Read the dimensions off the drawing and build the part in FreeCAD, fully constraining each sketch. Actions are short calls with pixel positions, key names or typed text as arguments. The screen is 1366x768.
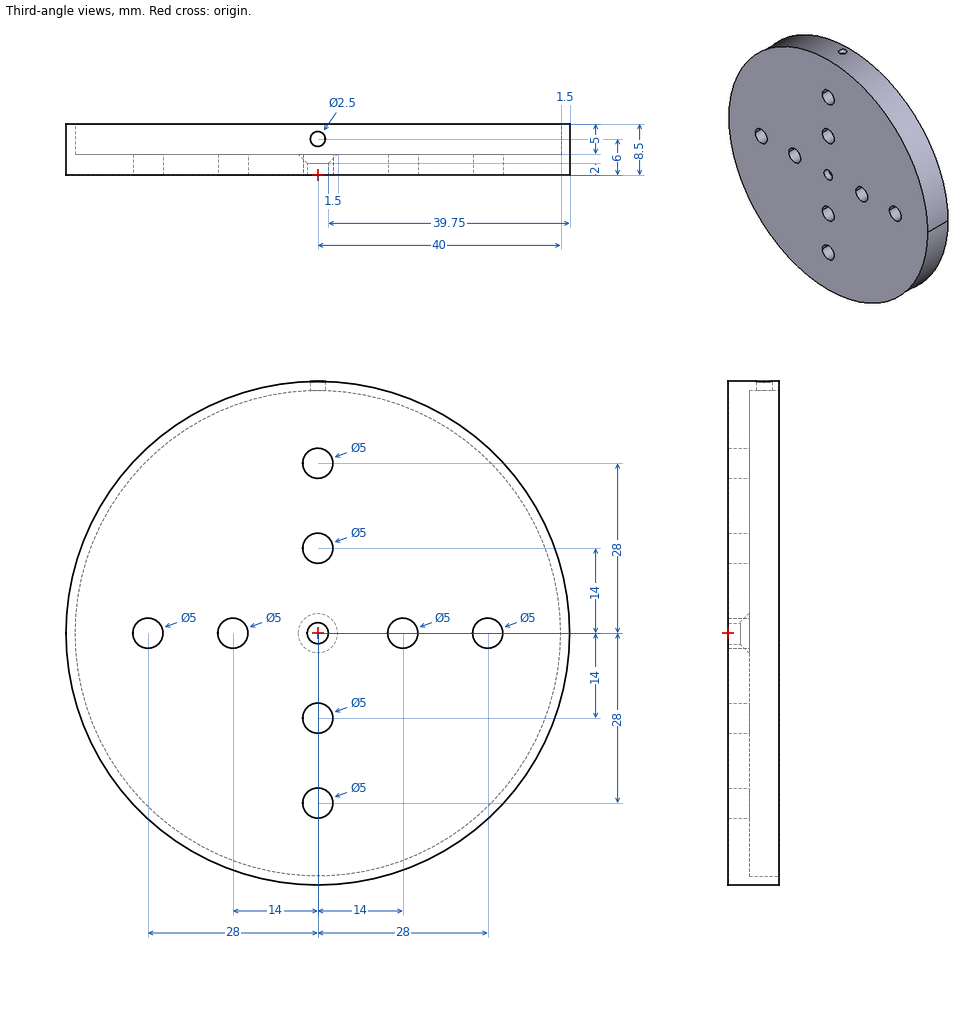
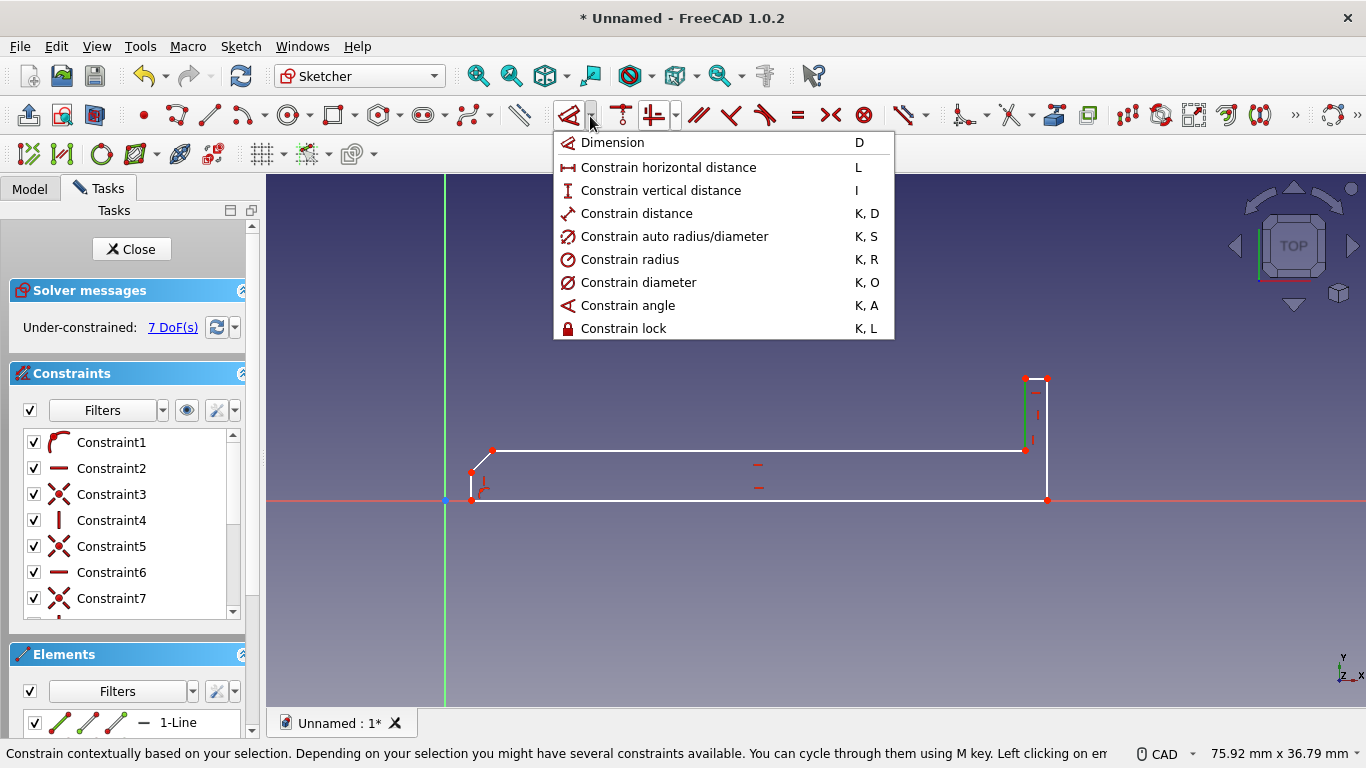
click(724, 190)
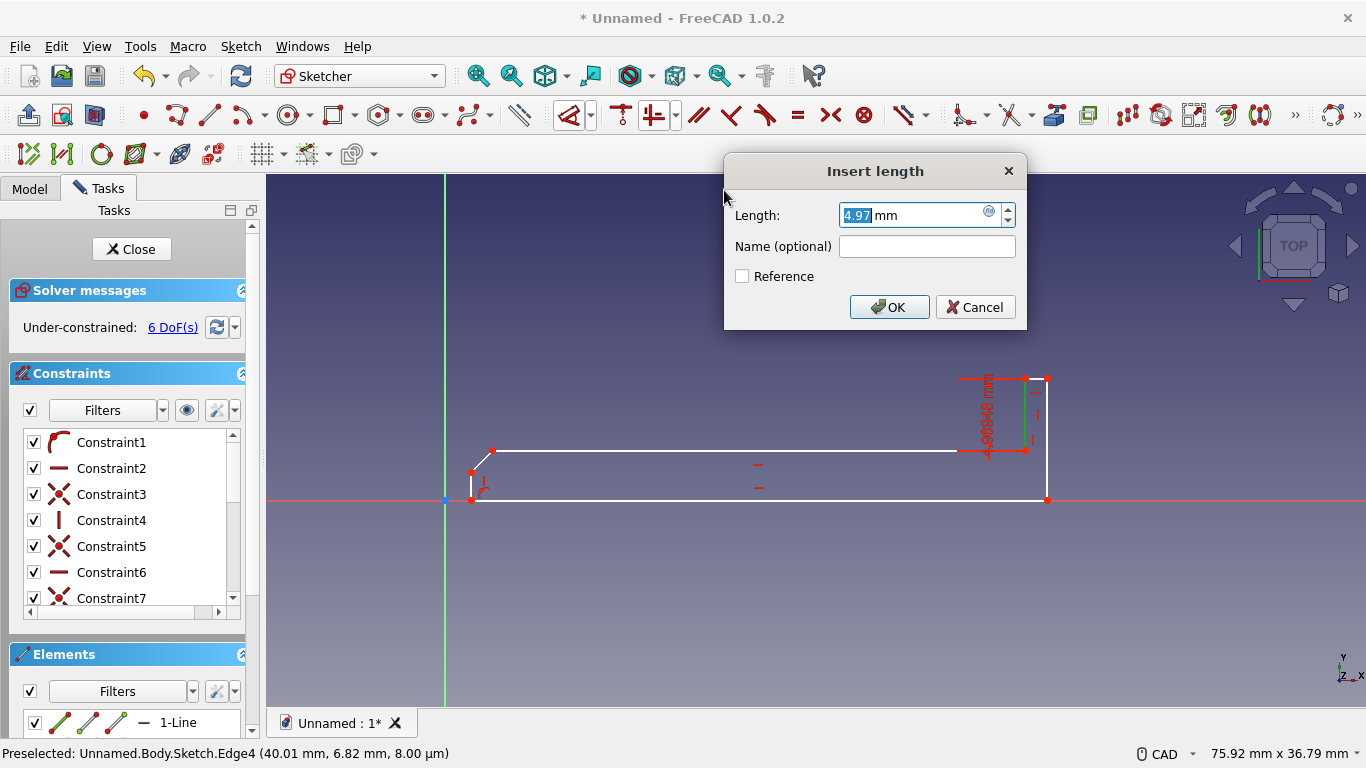
text(5)
key(Return)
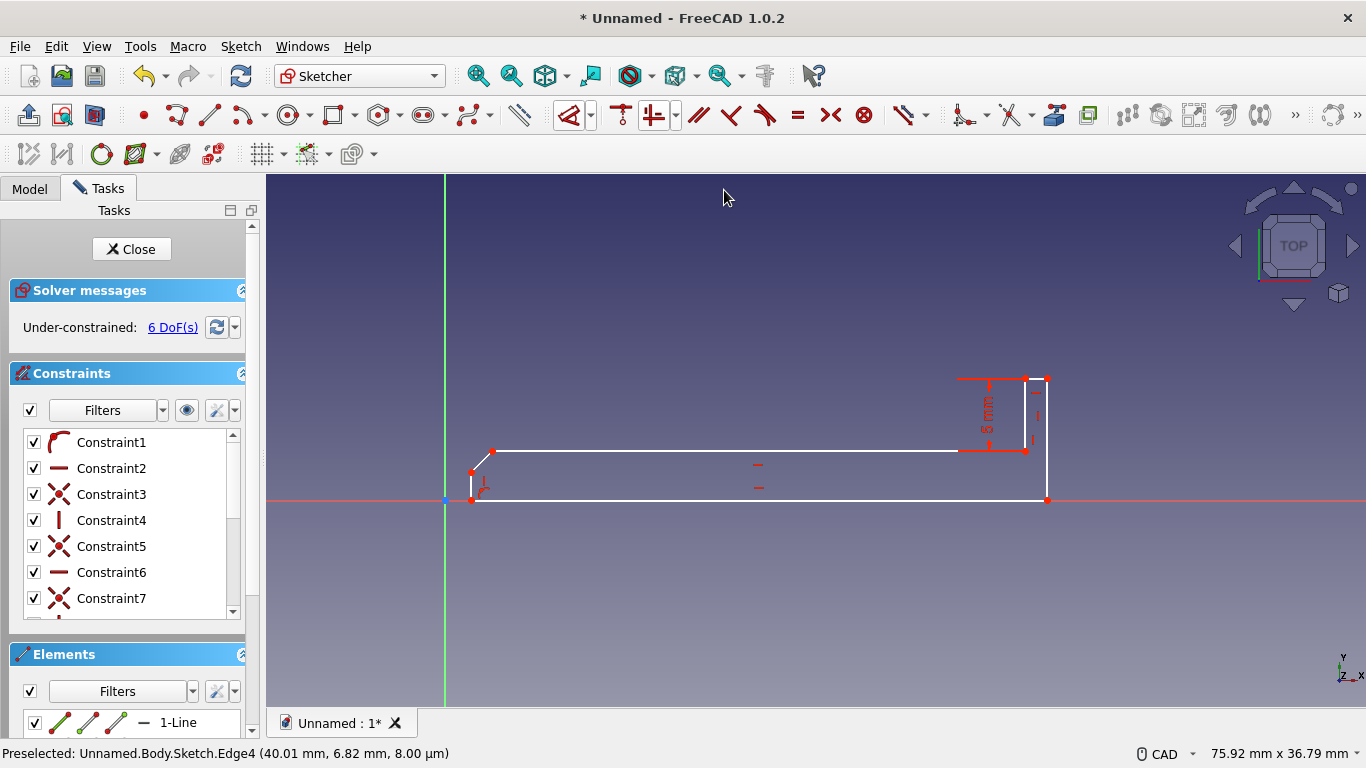
scroll(471, 484, up, 2)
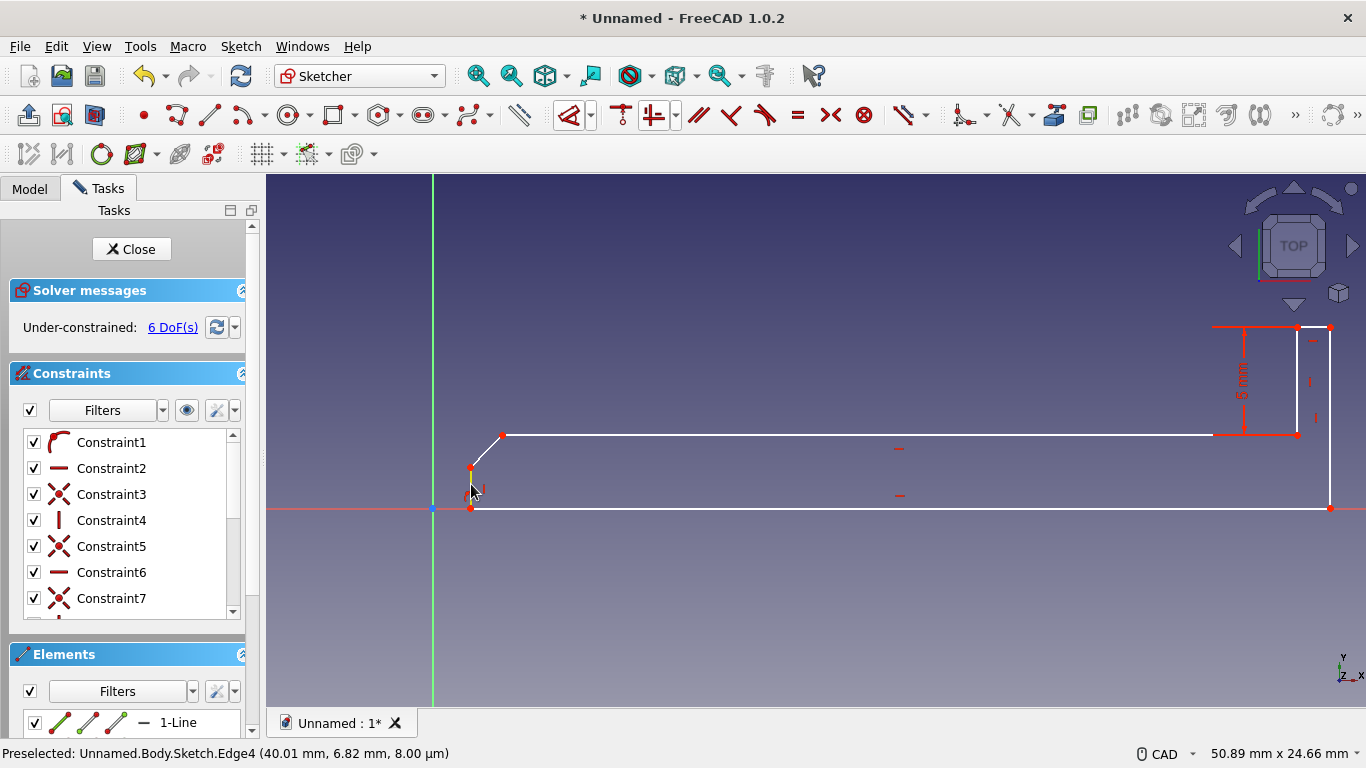
click(471, 484)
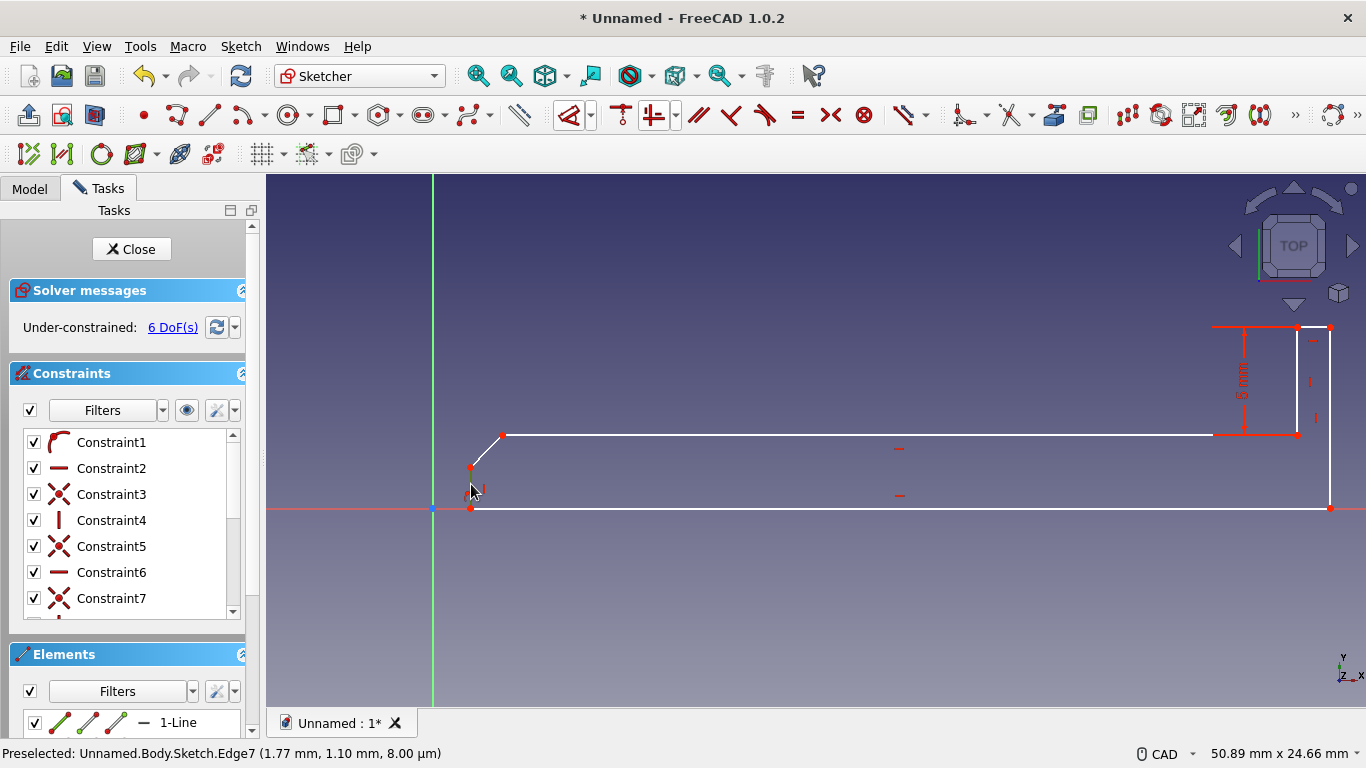
key(i)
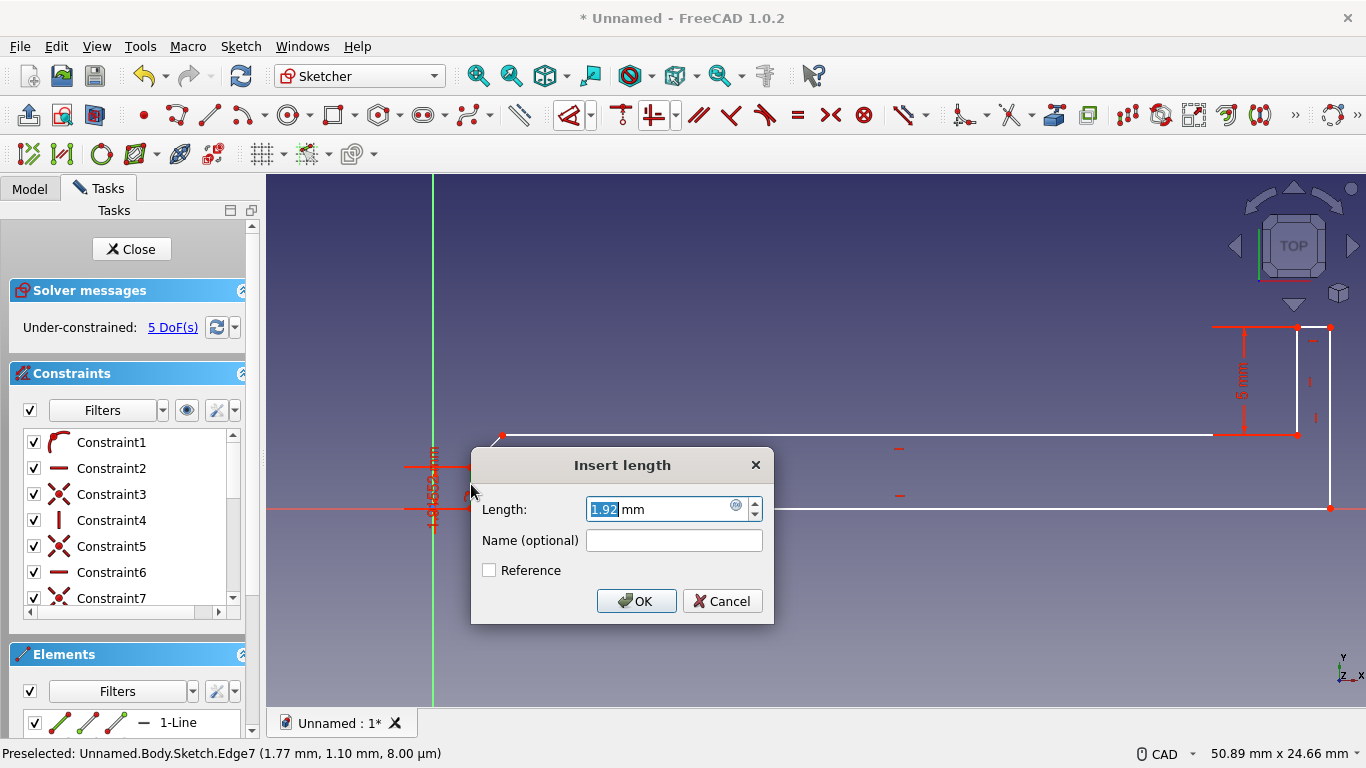
text(2)
key(Return)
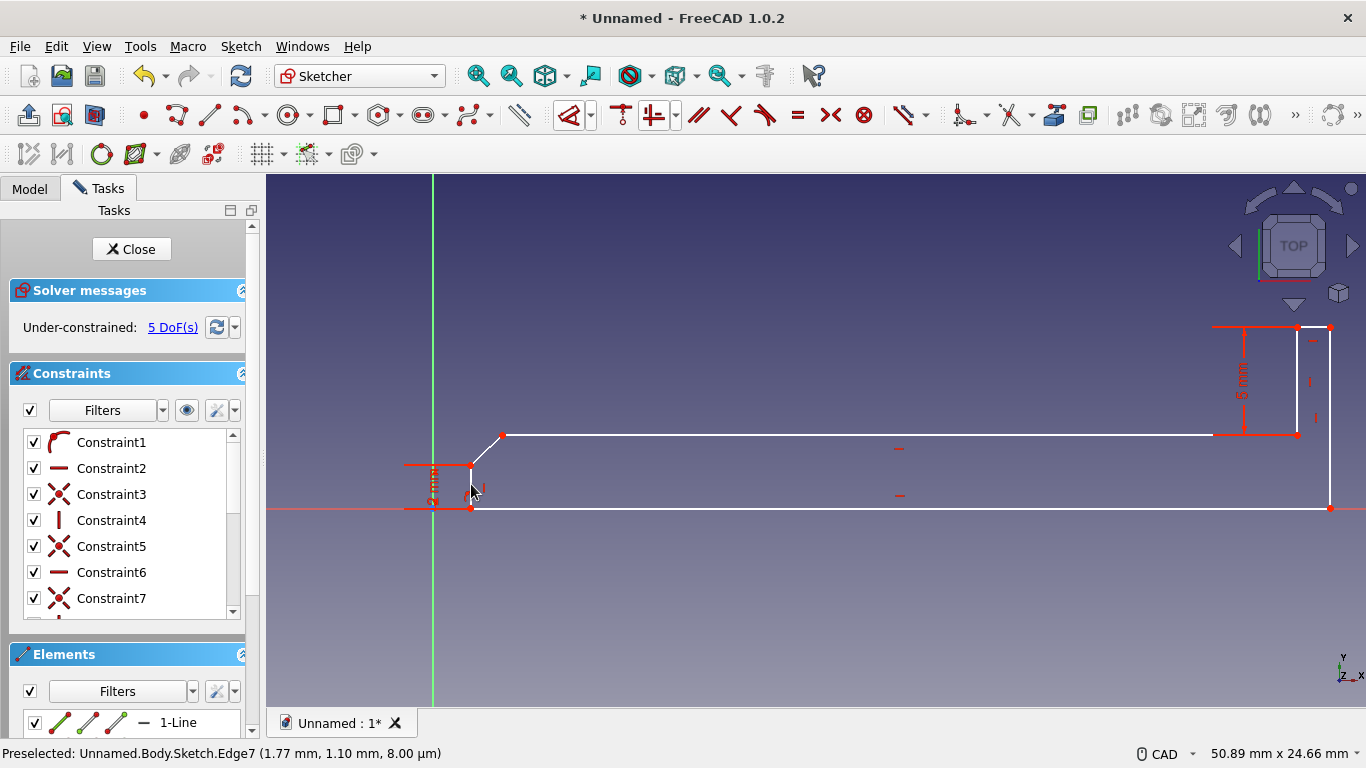
scroll(476, 489, down, 2)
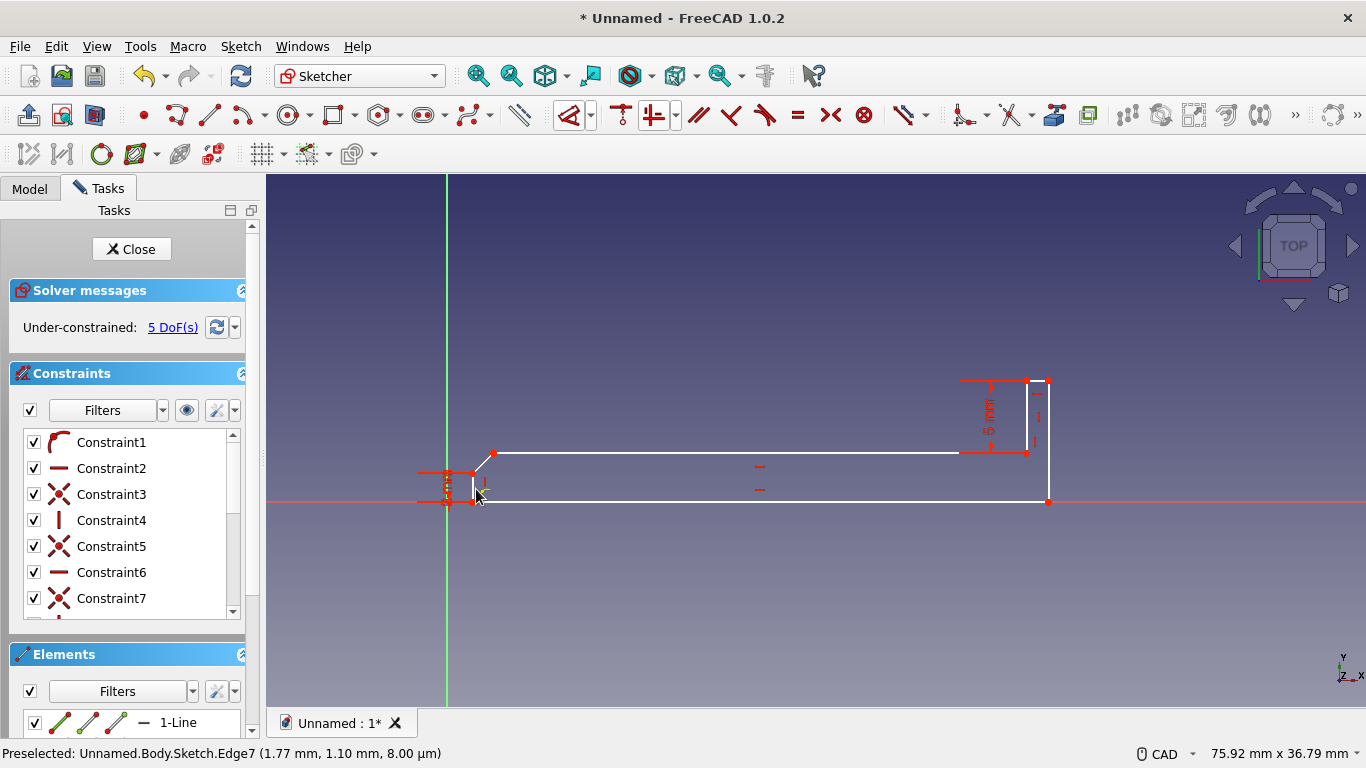
click(1049, 466)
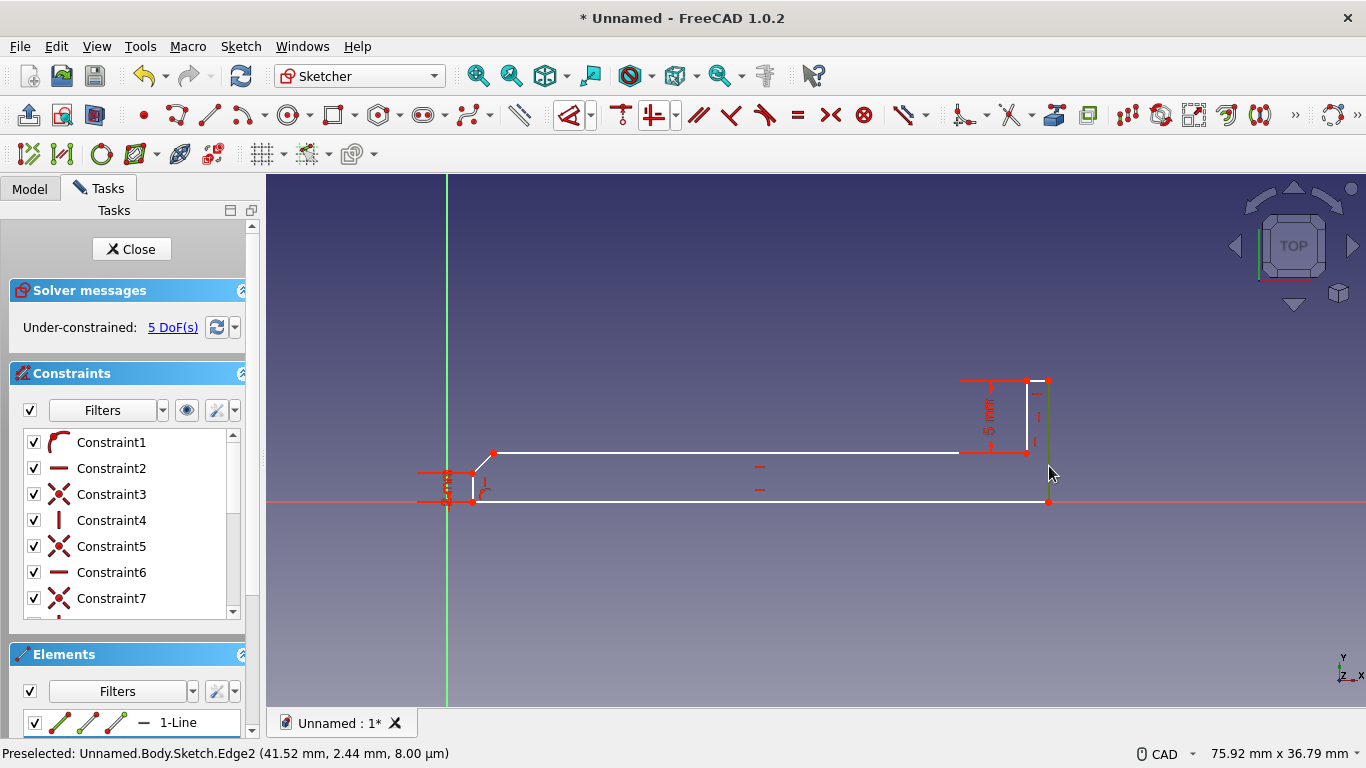
click(590, 116)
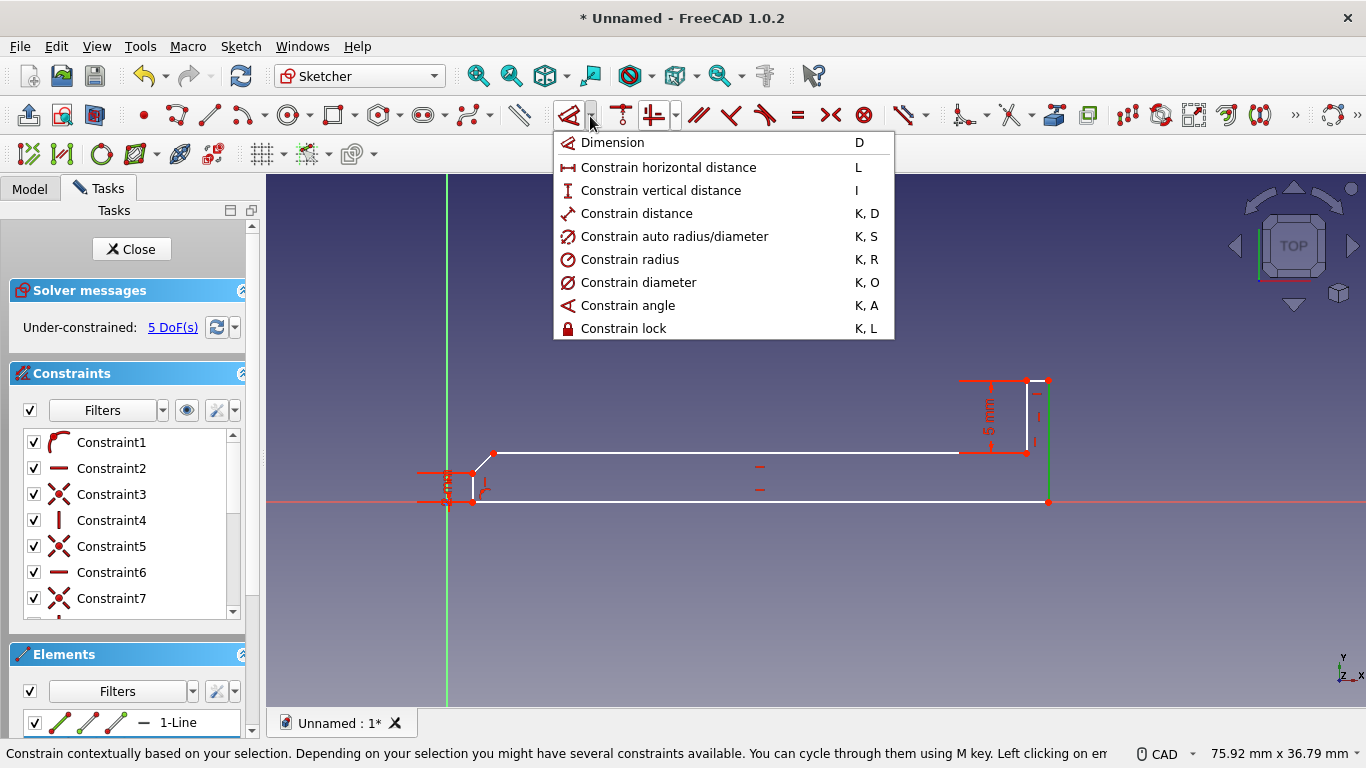
click(724, 190)